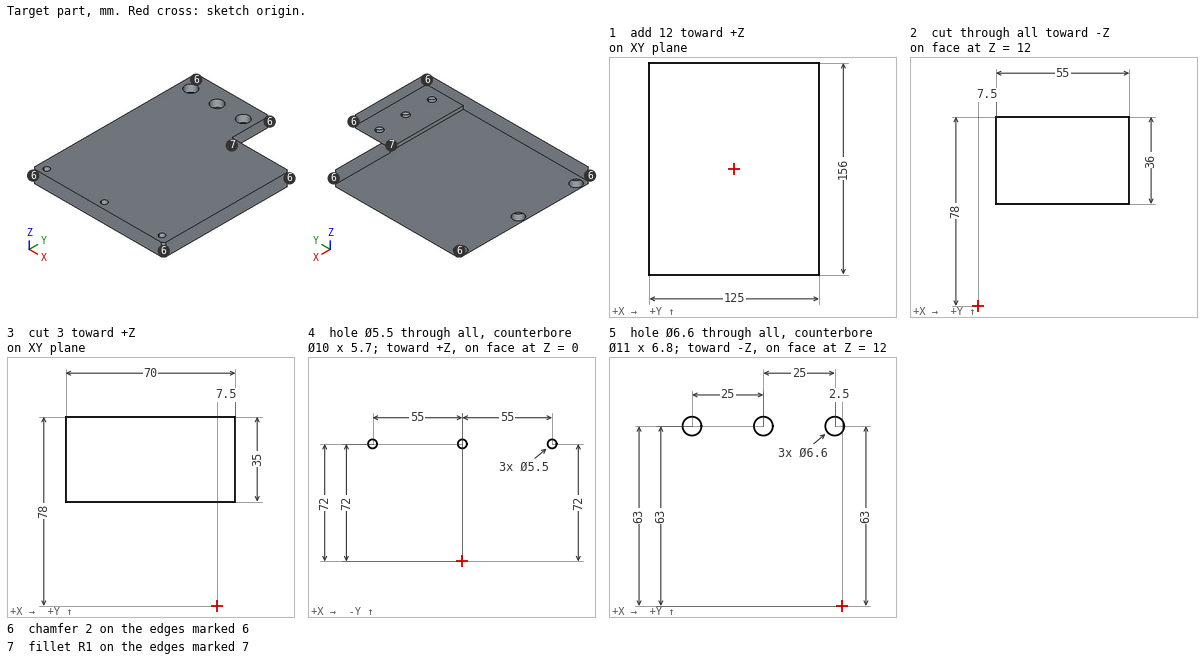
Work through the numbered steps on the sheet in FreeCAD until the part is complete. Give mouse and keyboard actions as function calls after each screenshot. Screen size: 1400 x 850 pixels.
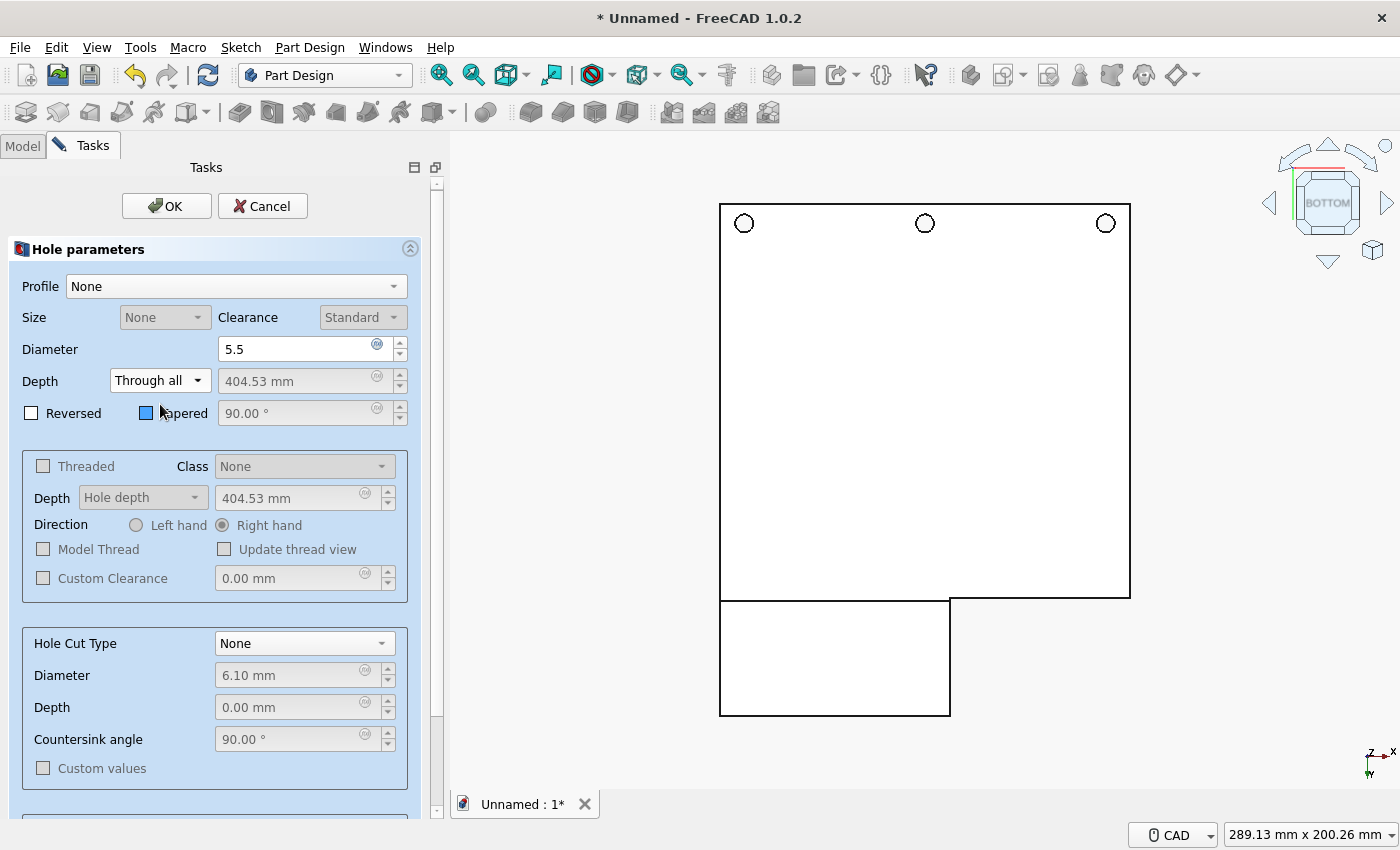
click(306, 644)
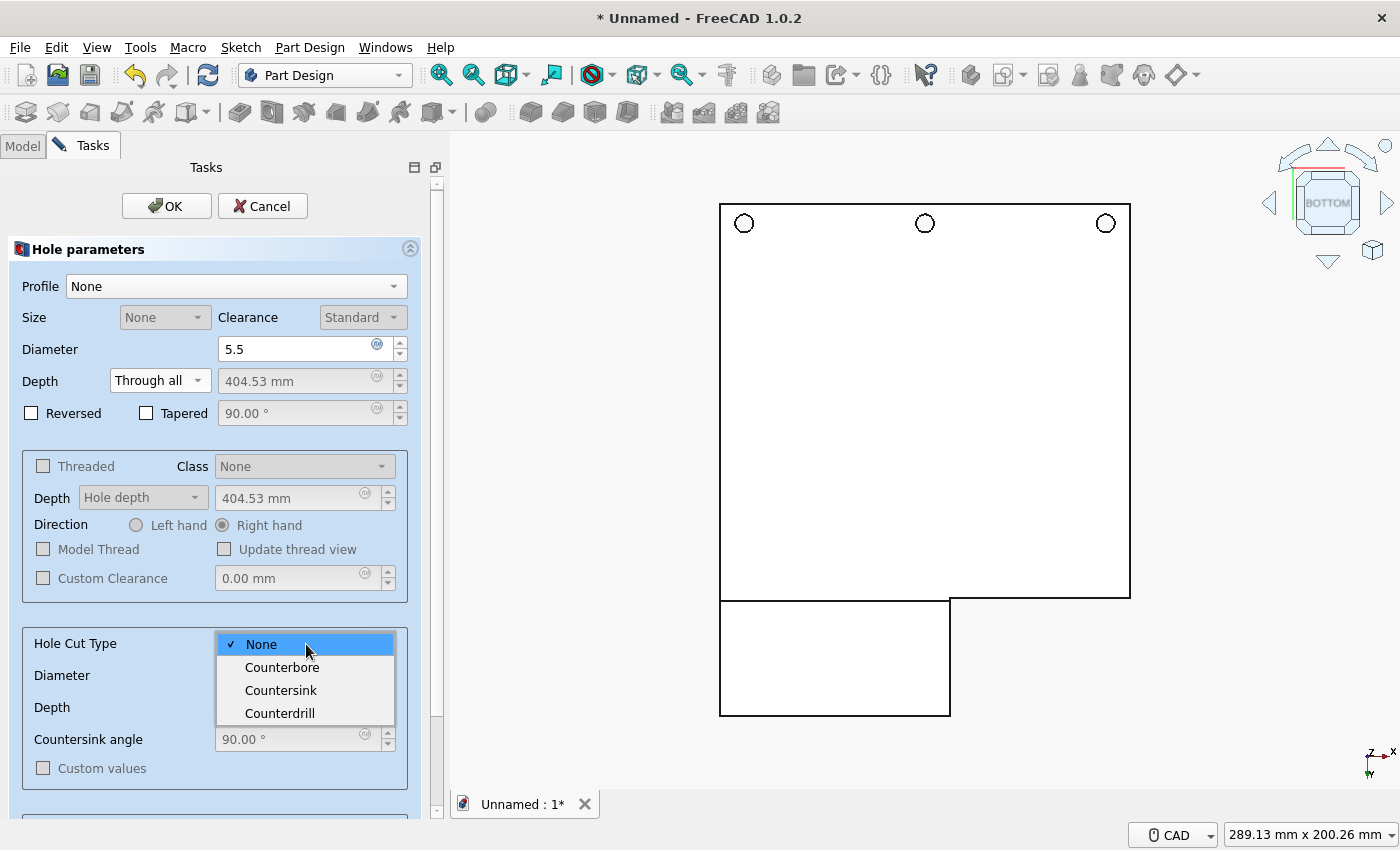
click(304, 668)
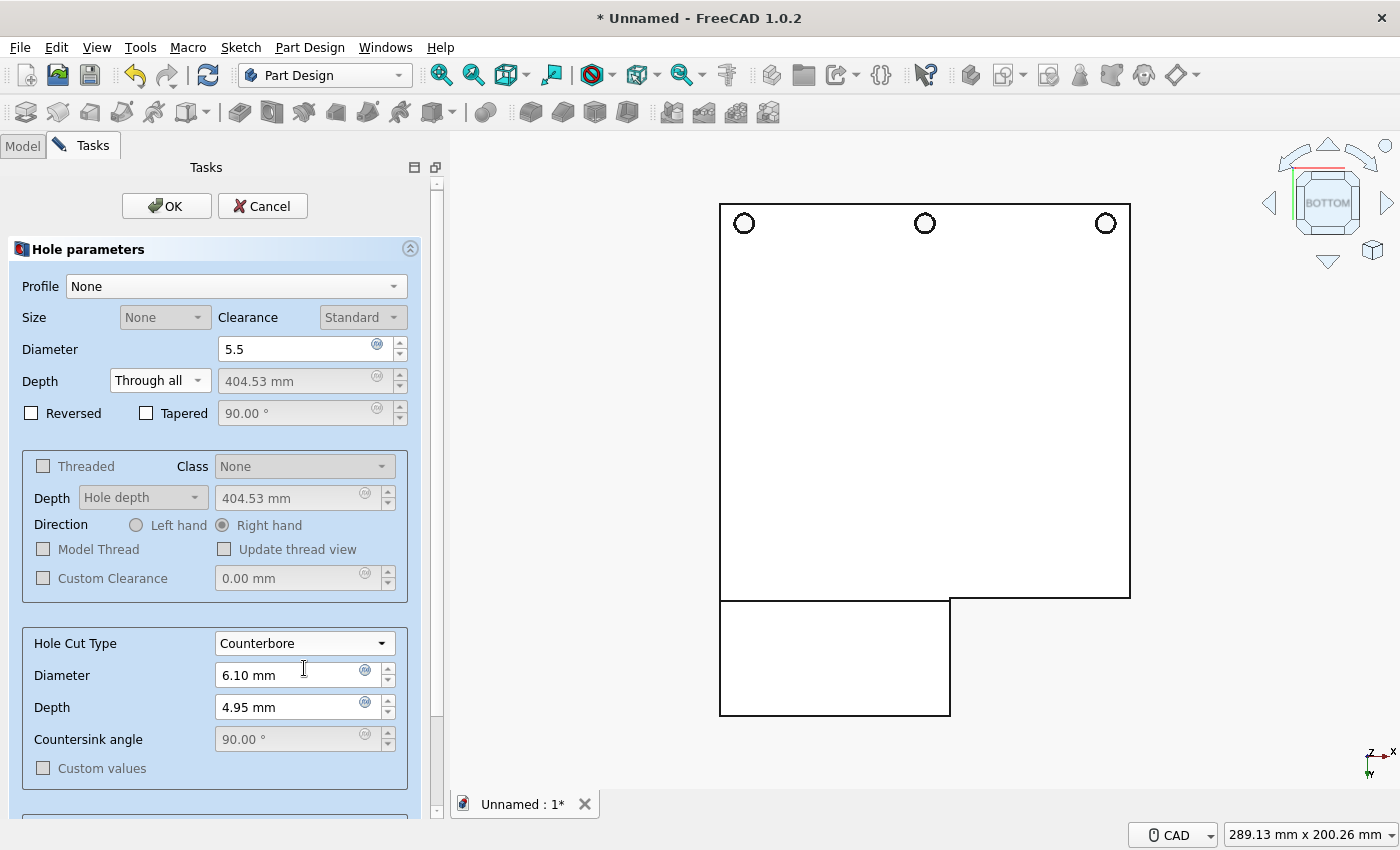
triple_click(298, 675)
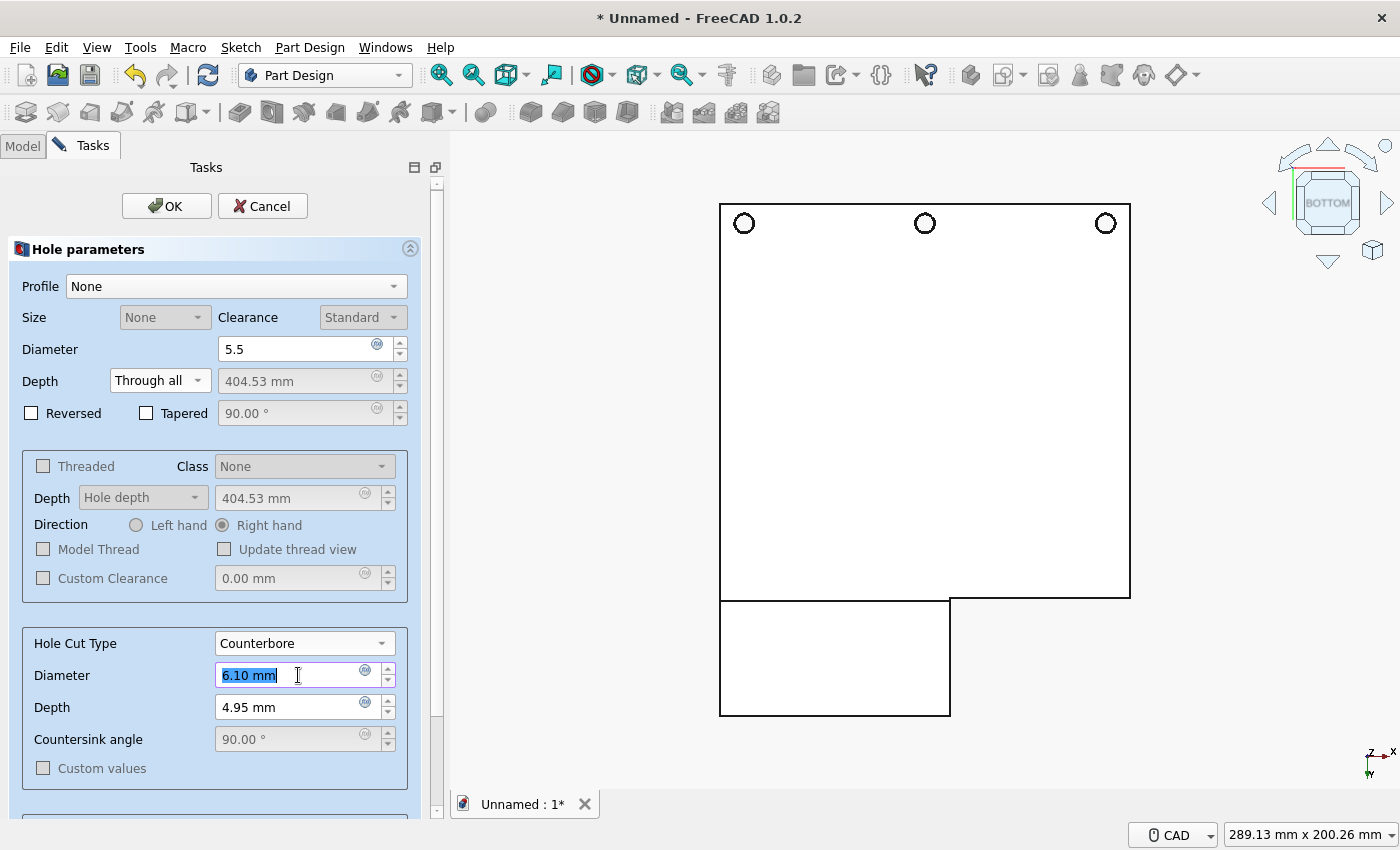
text(10)
key(Tab)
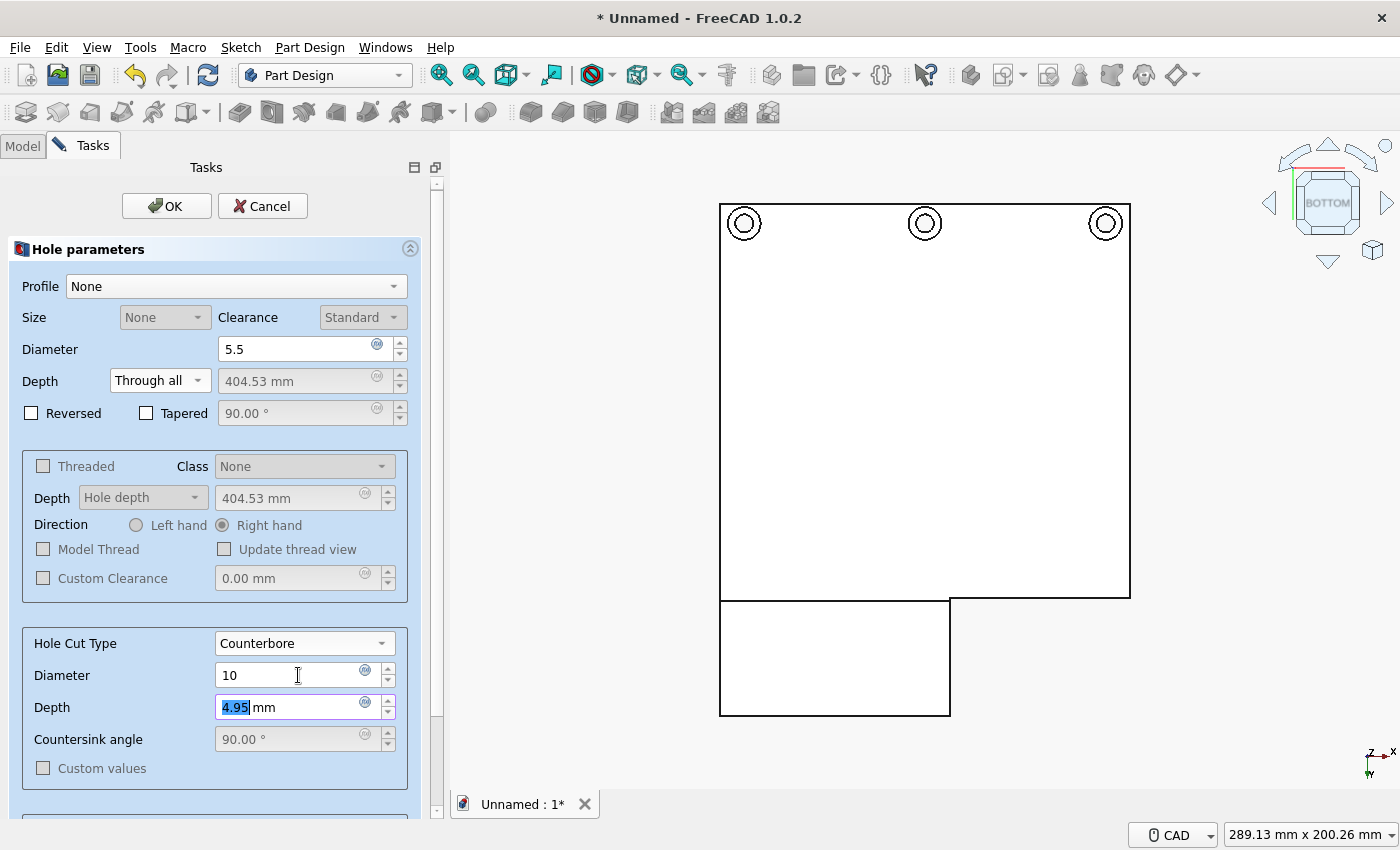
text(5.7)
key(Tab)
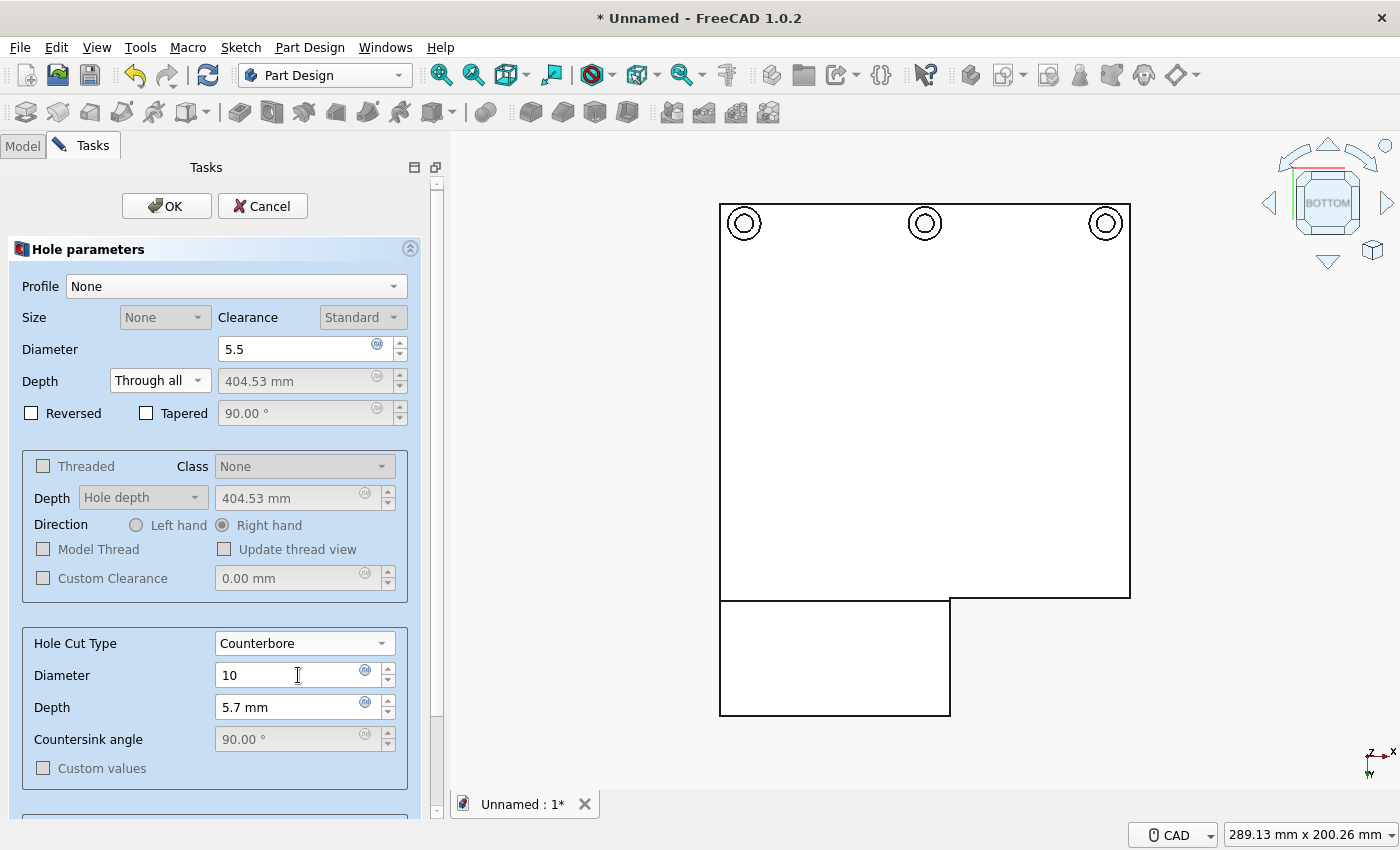
click(167, 206)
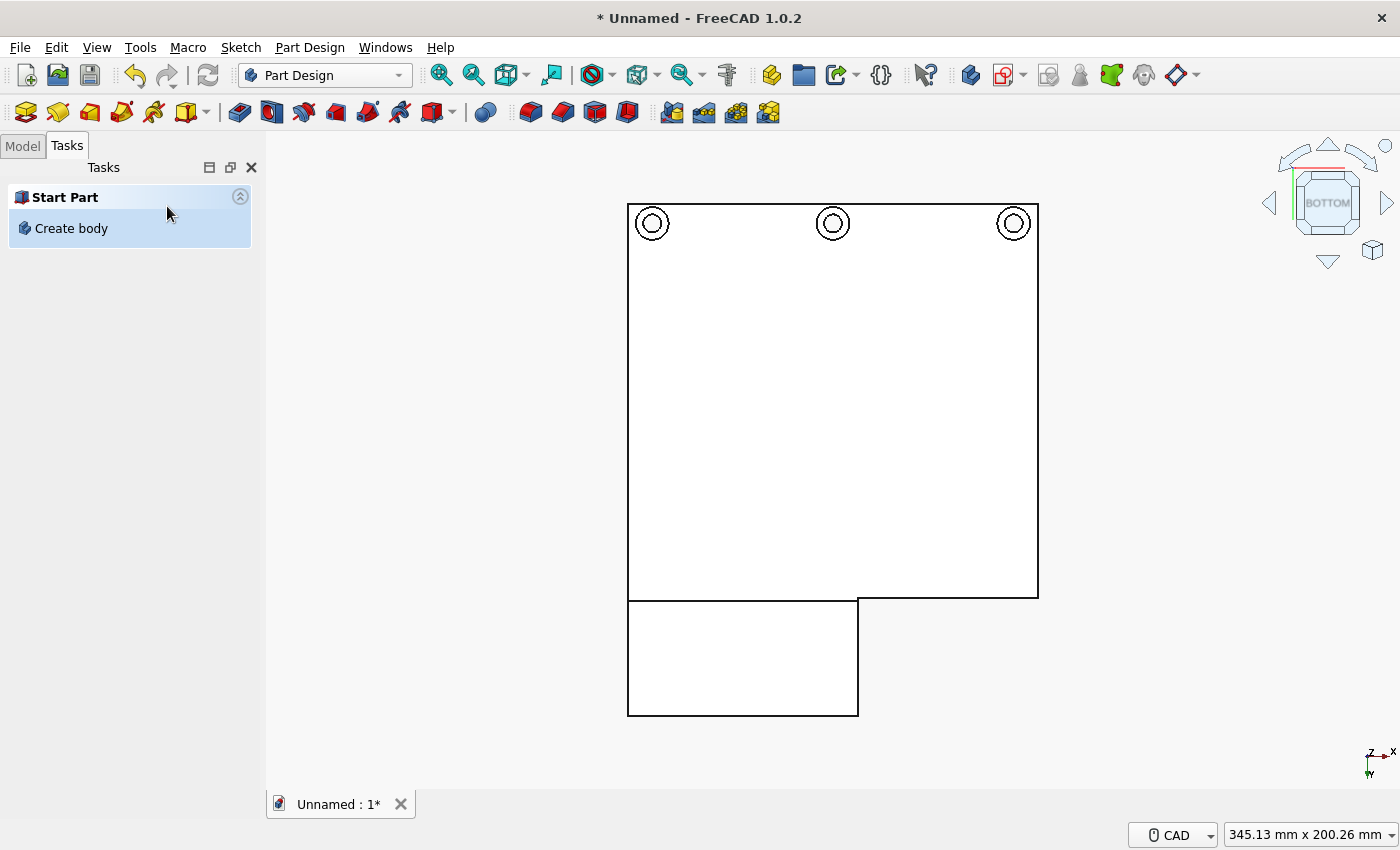
key(0)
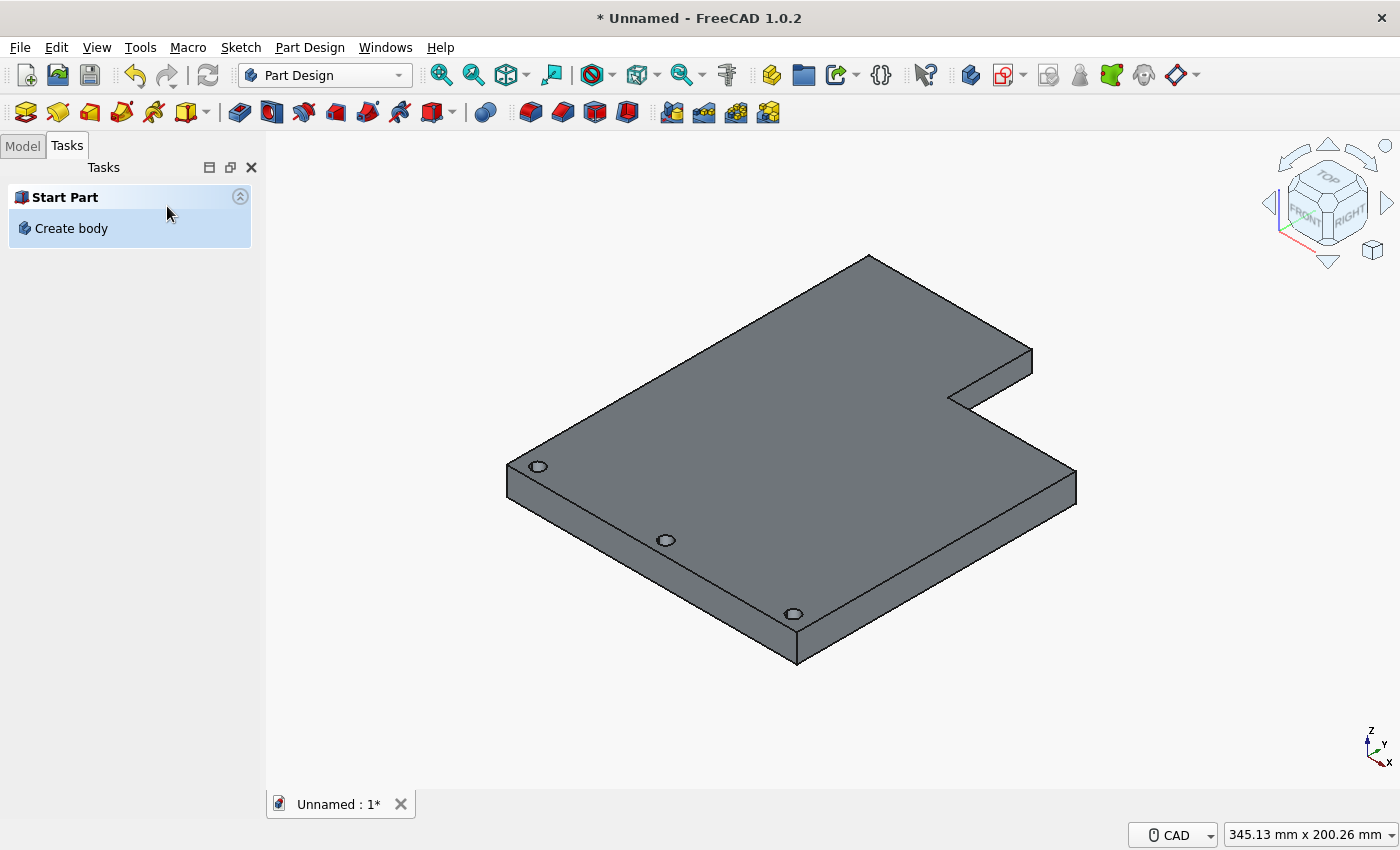
click(781, 473)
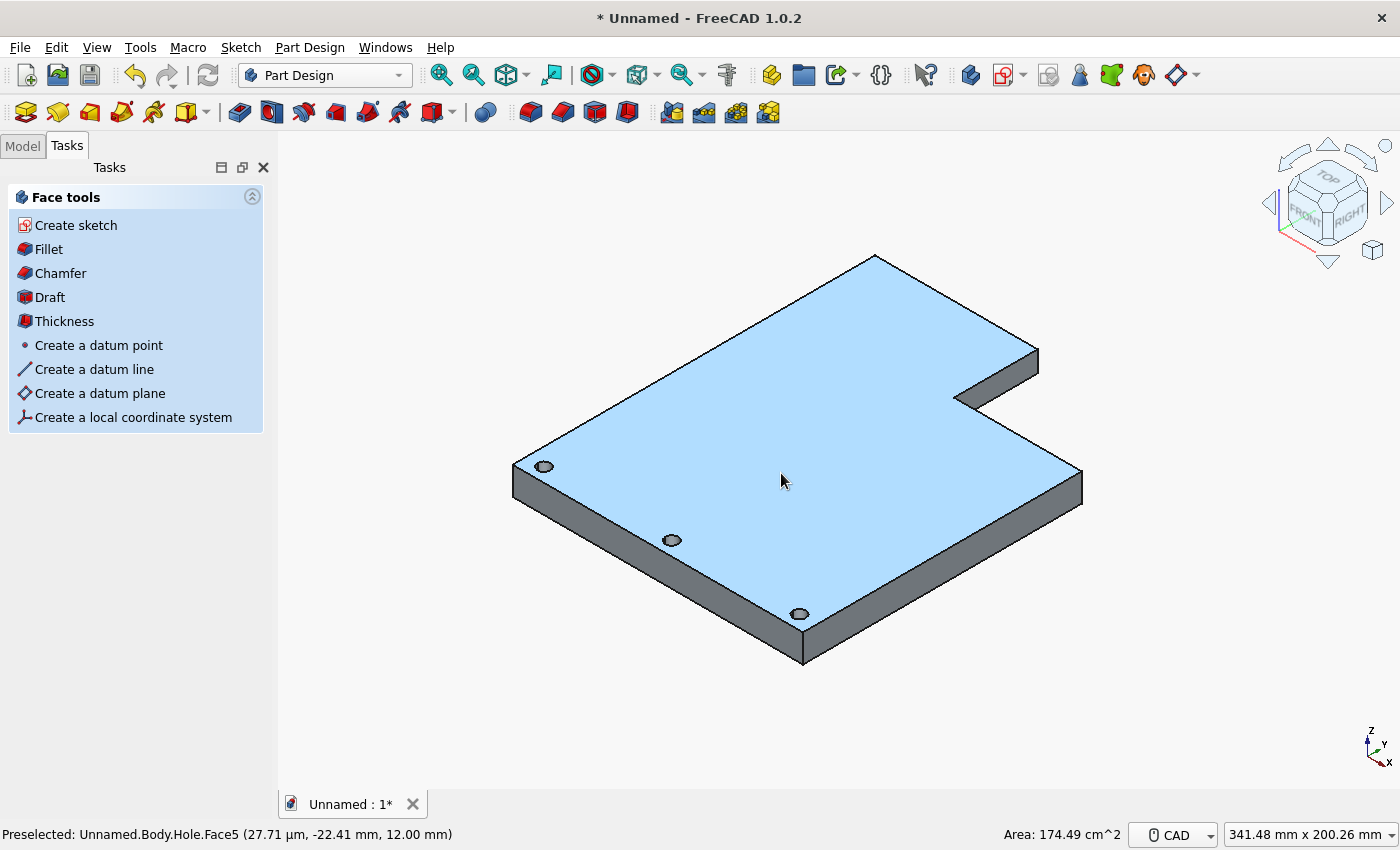
click(1004, 76)